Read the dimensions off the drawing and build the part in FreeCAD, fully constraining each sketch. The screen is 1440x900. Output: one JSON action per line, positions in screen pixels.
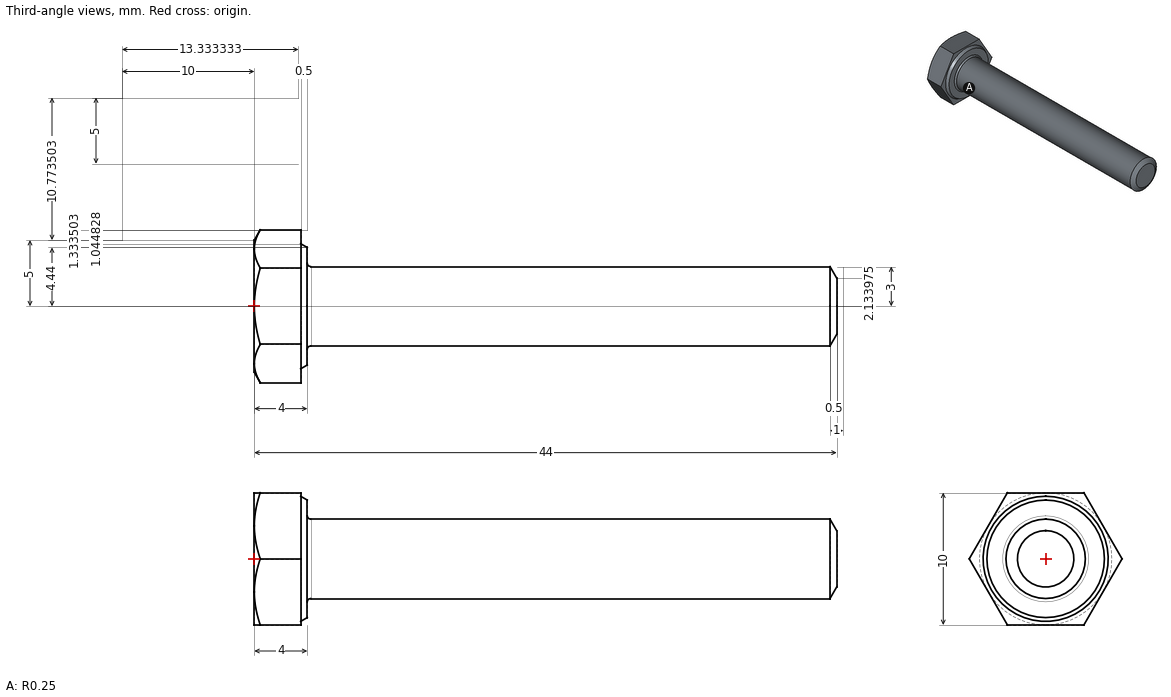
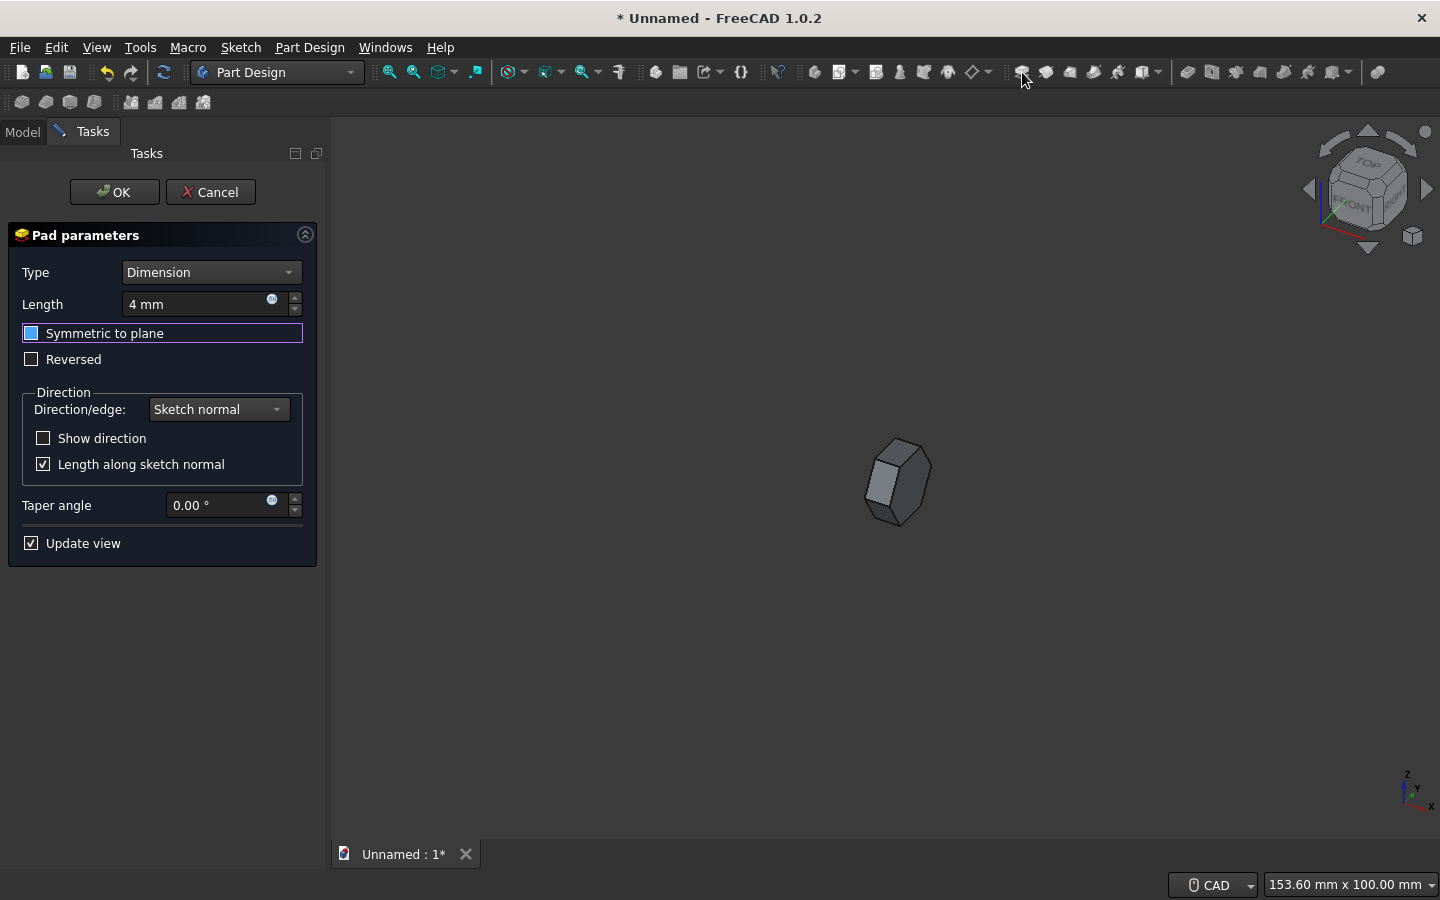
{"action": "left_click", "coordinate": [115, 192]}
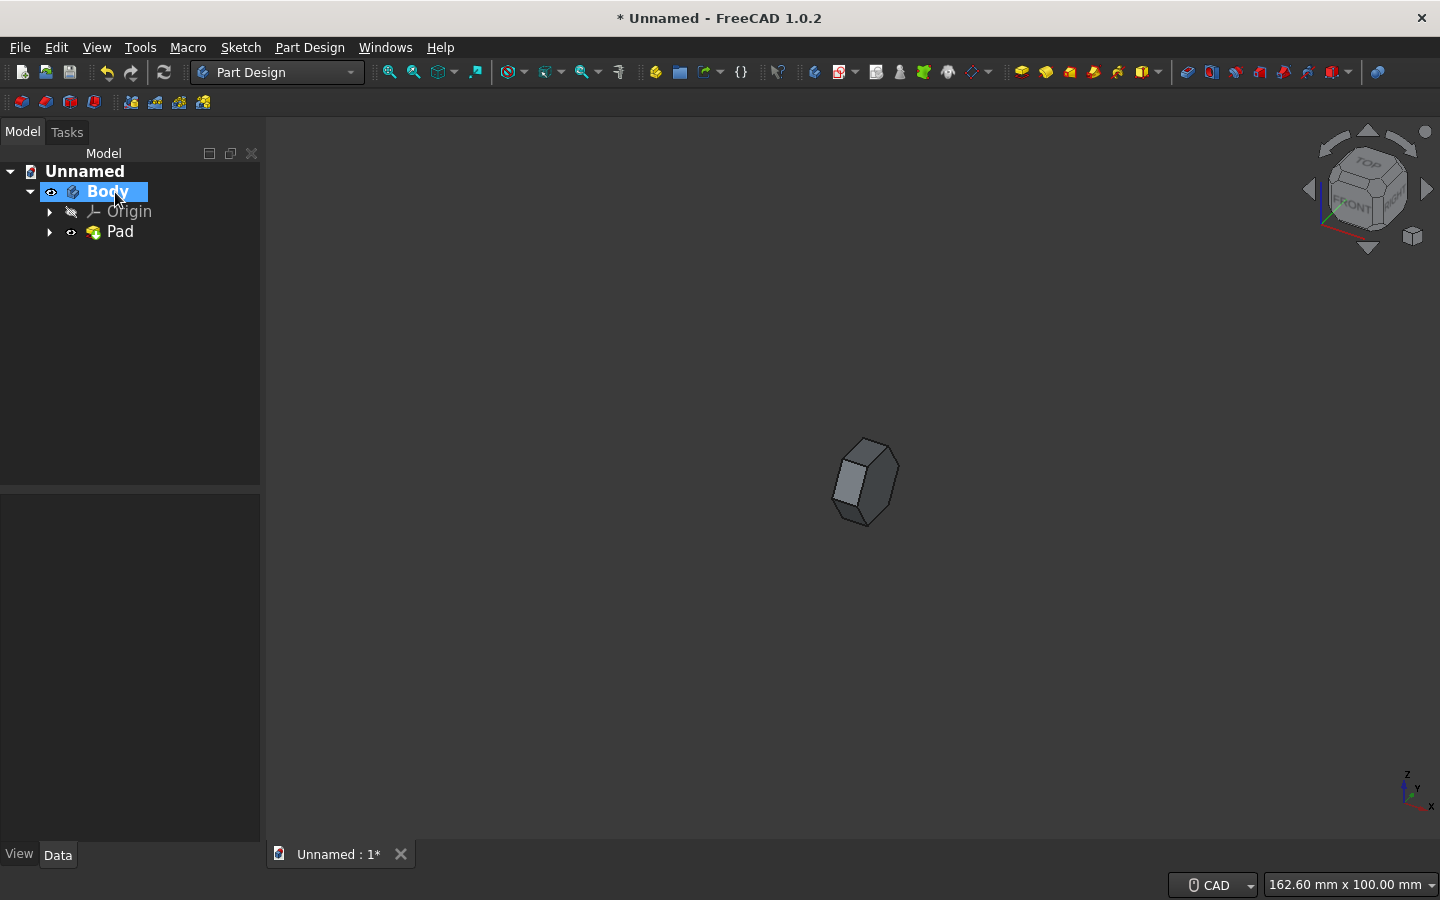
{"action": "left_click", "coordinate": [390, 72]}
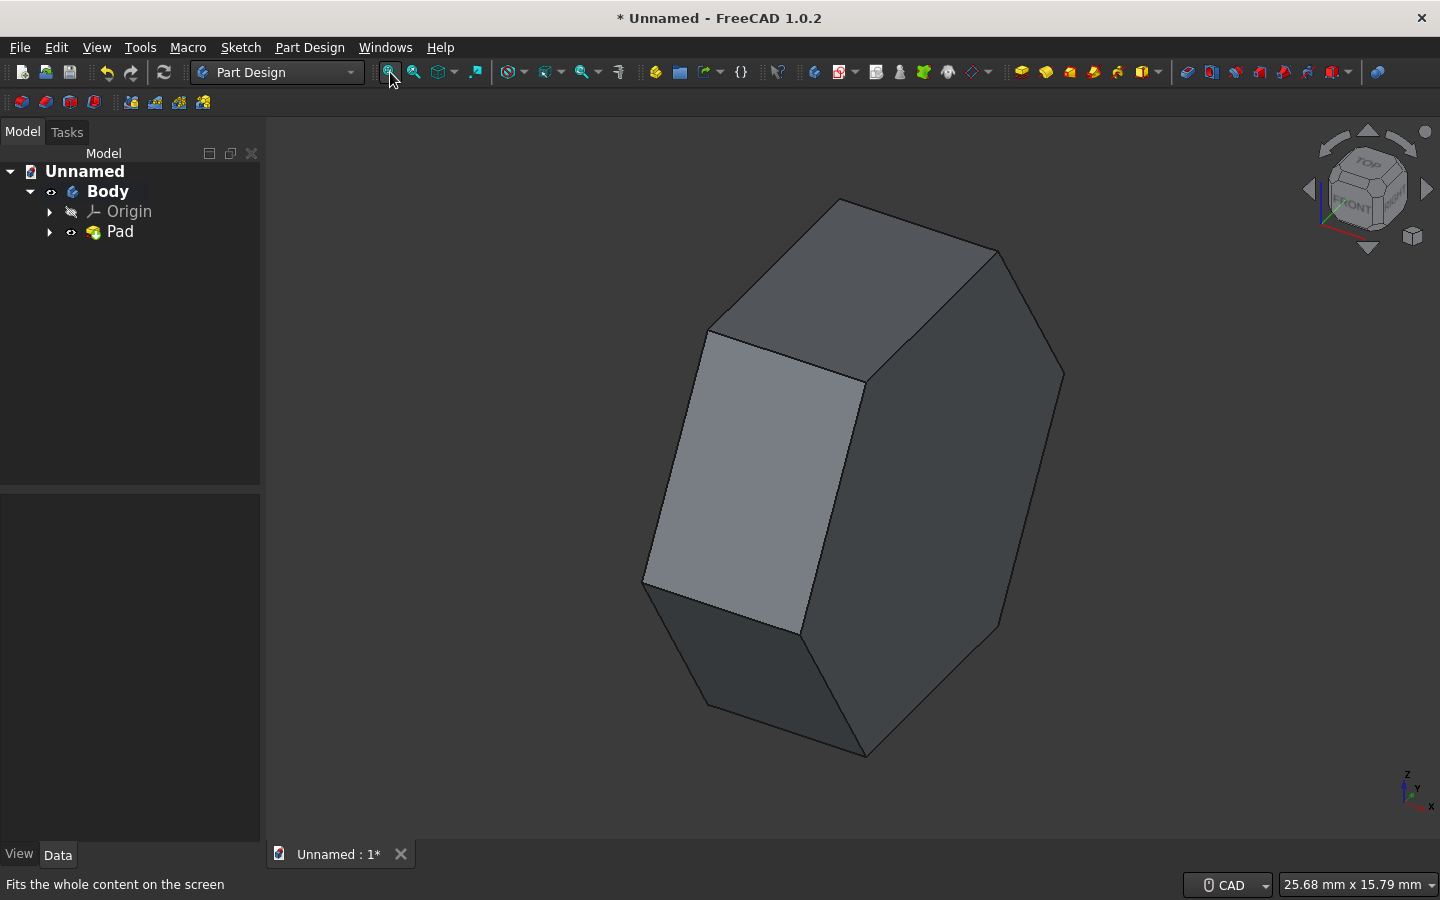
{"action": "left_click", "coordinate": [840, 72]}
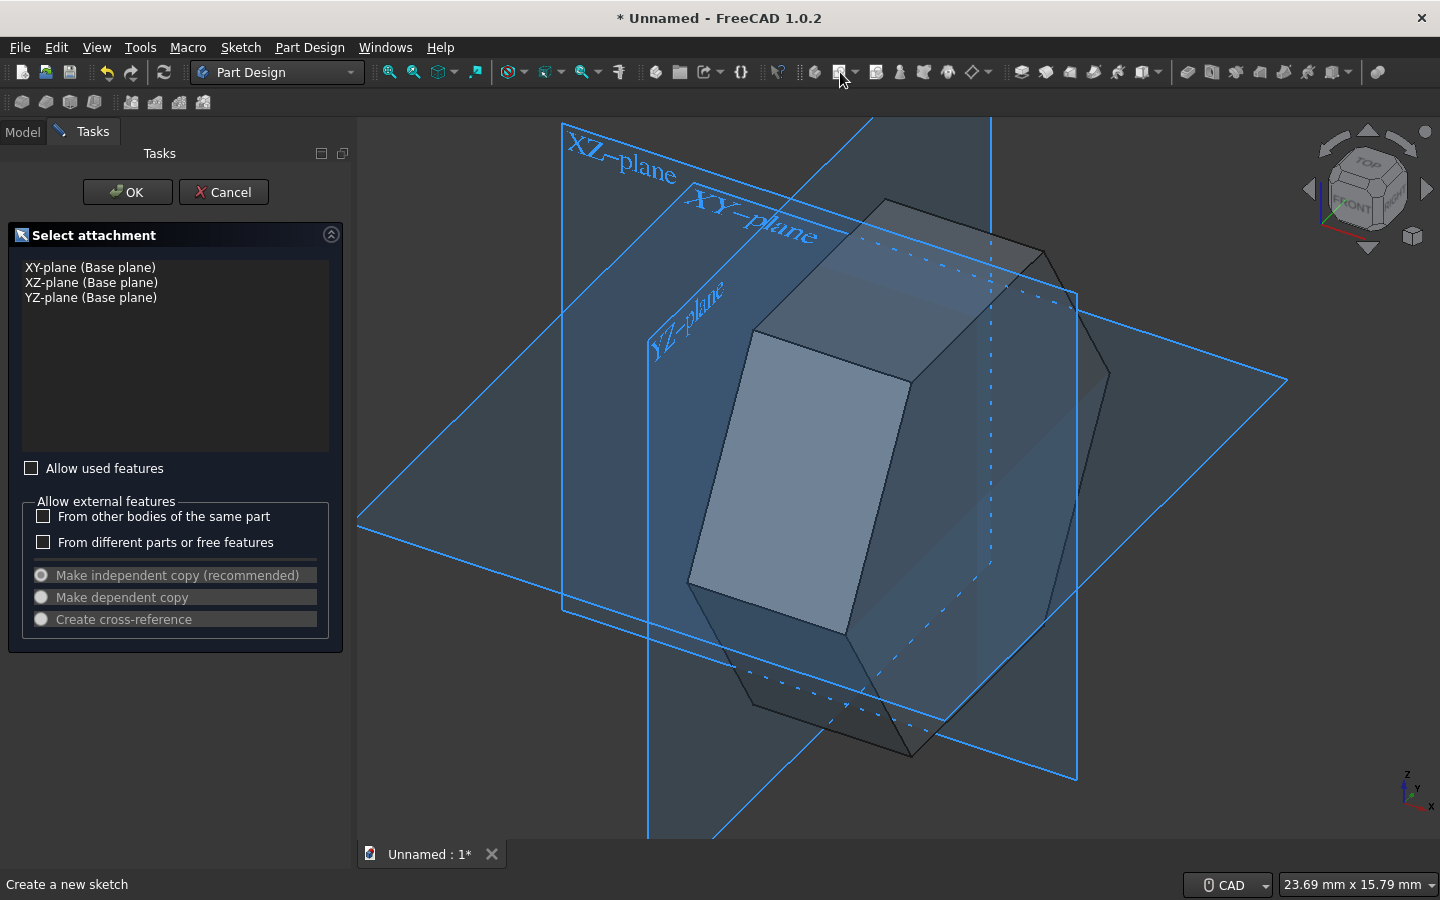
{"action": "left_click", "coordinate": [82, 268]}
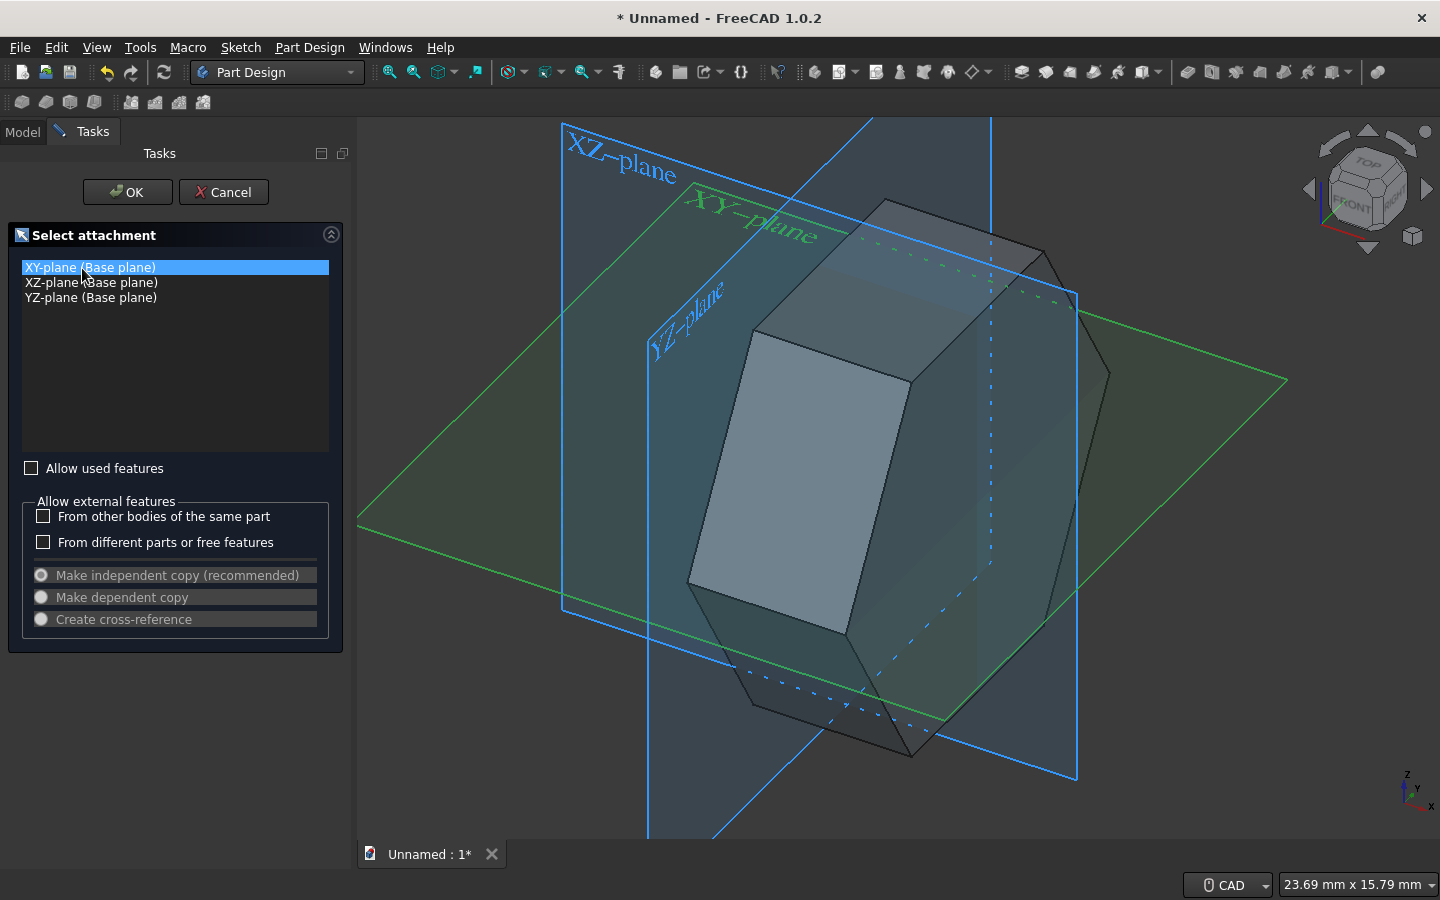
{"action": "left_click", "coordinate": [128, 192]}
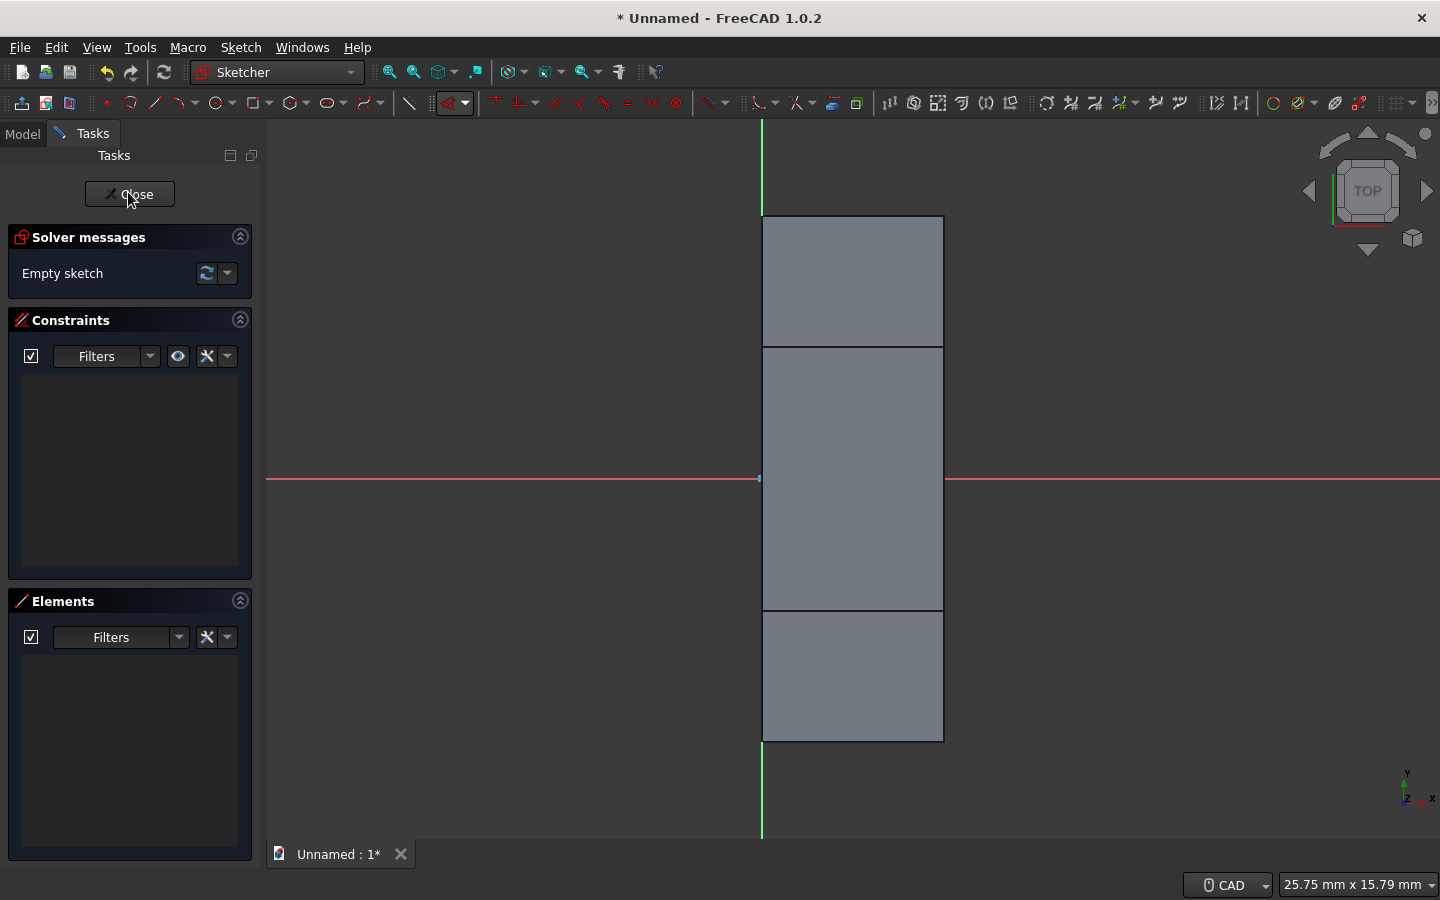
{"action": "left_click", "coordinate": [70, 104]}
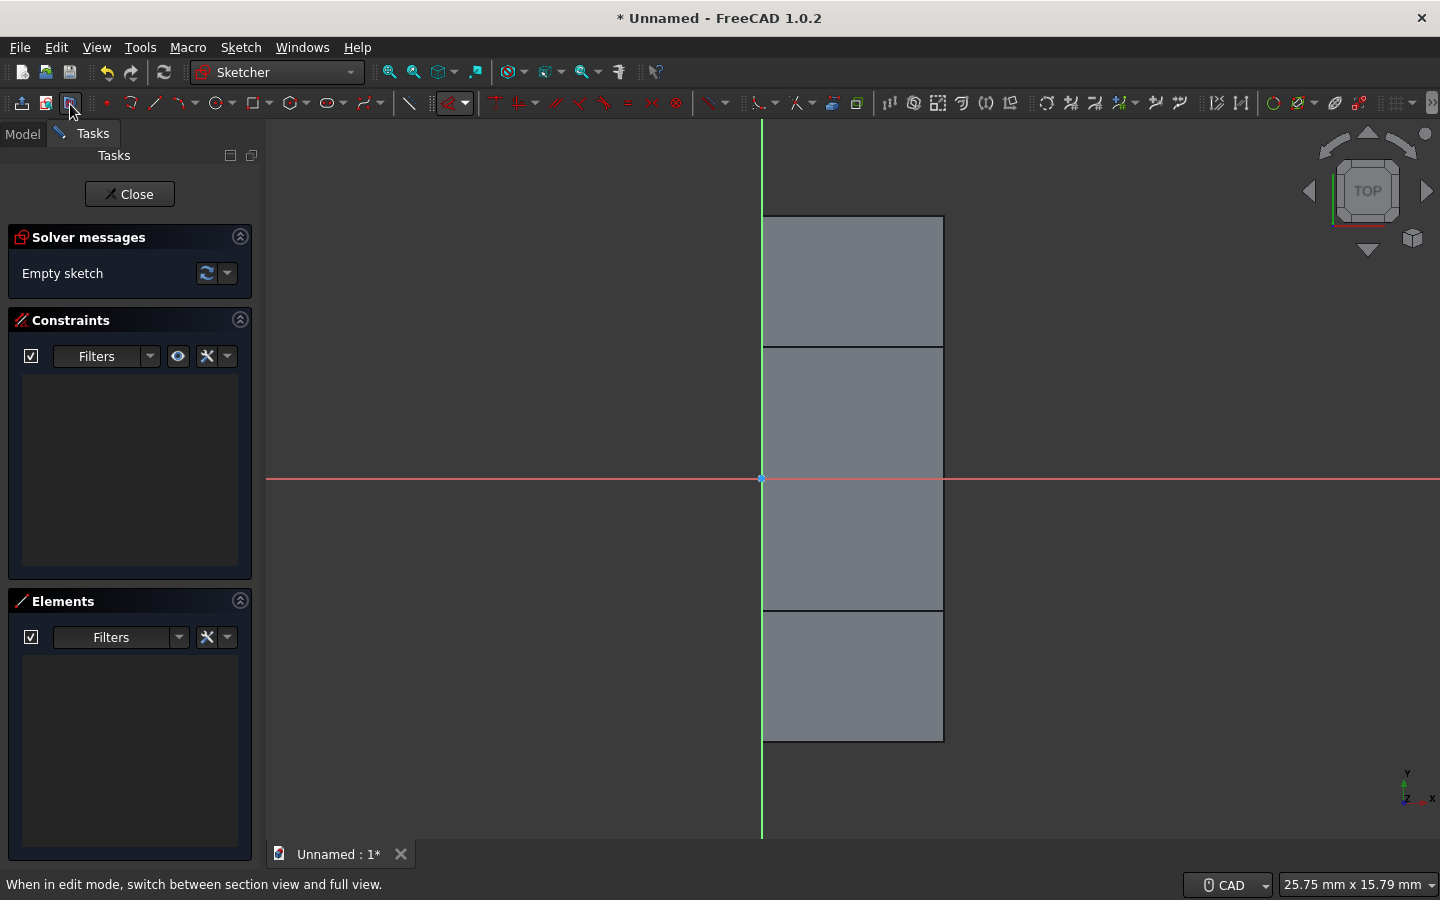
{"action": "scroll", "coordinate": [294, 519], "scroll_direction": "down", "scroll_amount": 5}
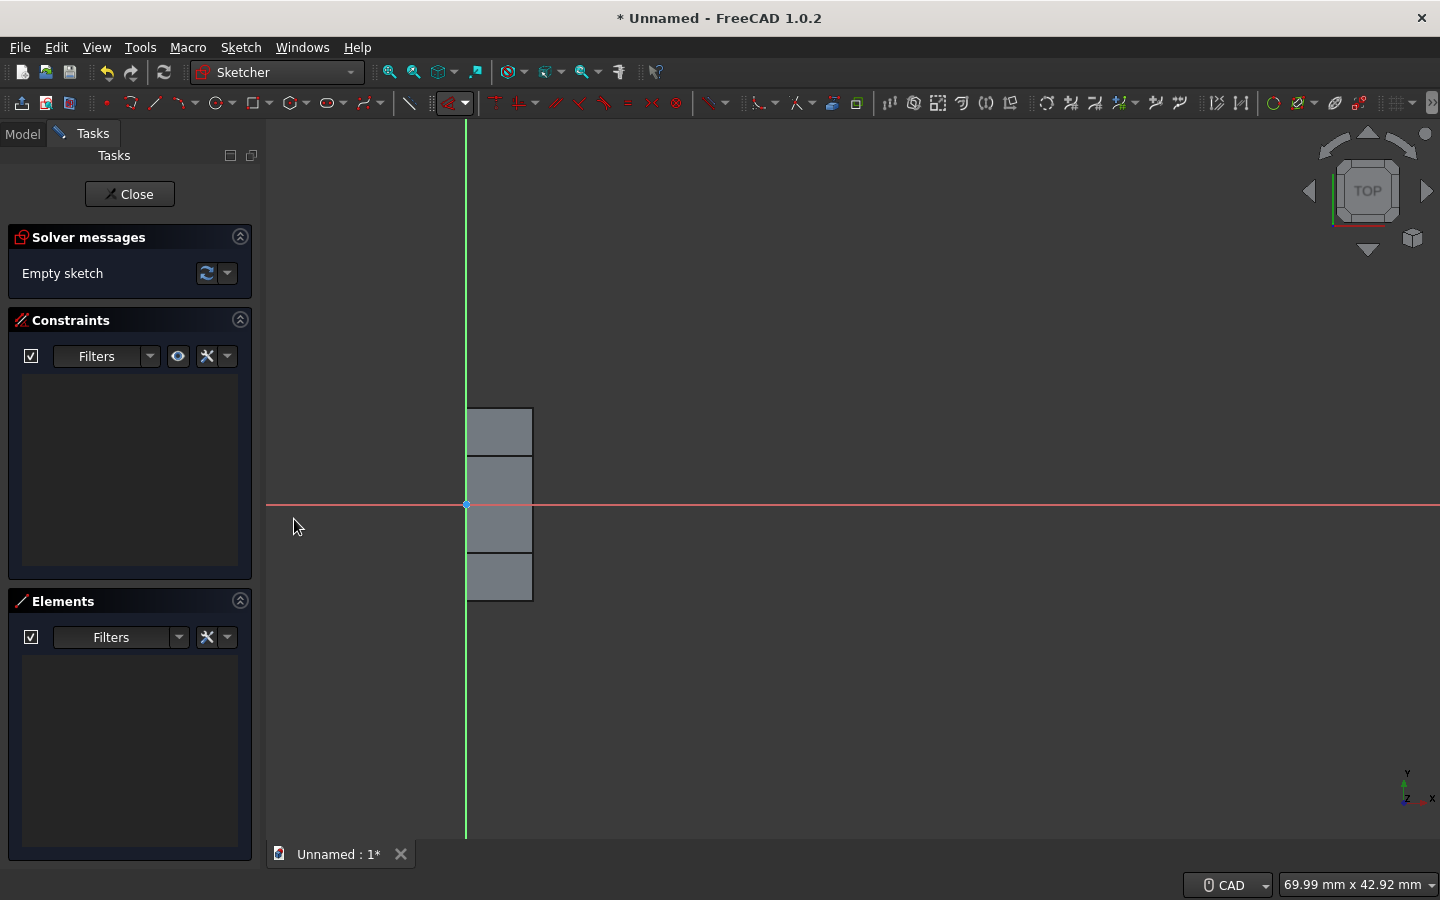
{"action": "left_click", "coordinate": [254, 104]}